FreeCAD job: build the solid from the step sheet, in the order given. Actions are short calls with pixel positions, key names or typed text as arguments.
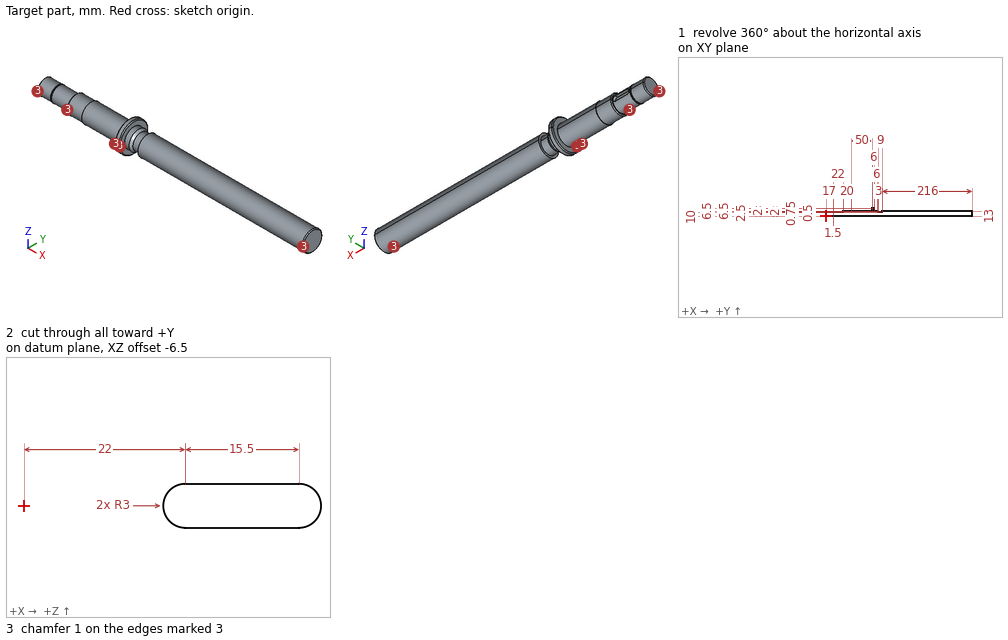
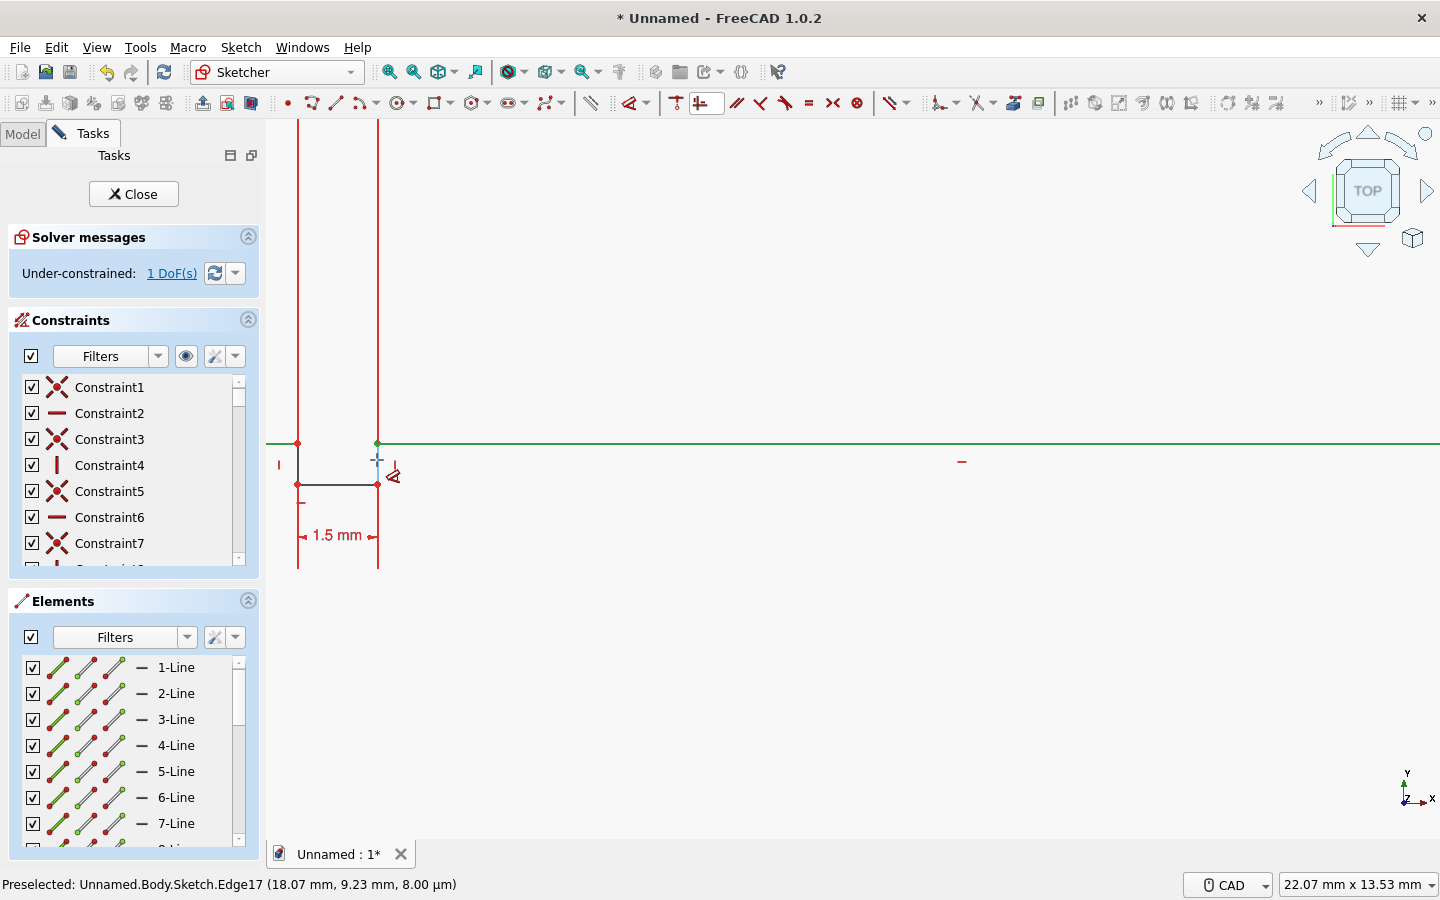
click(378, 460)
click(344, 464)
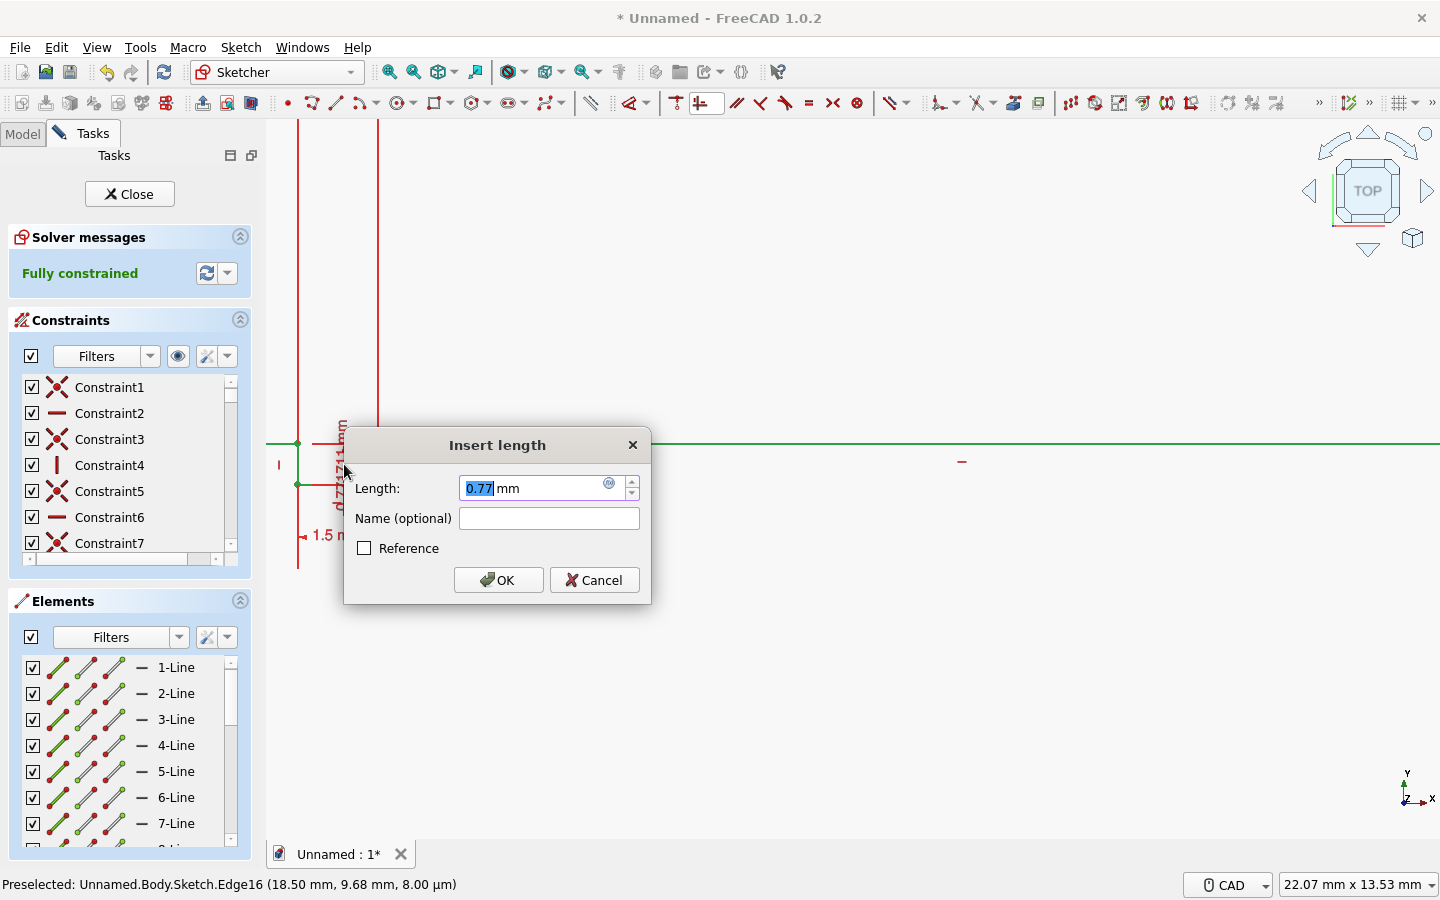
text(0.75)
key(Return)
key(Escape)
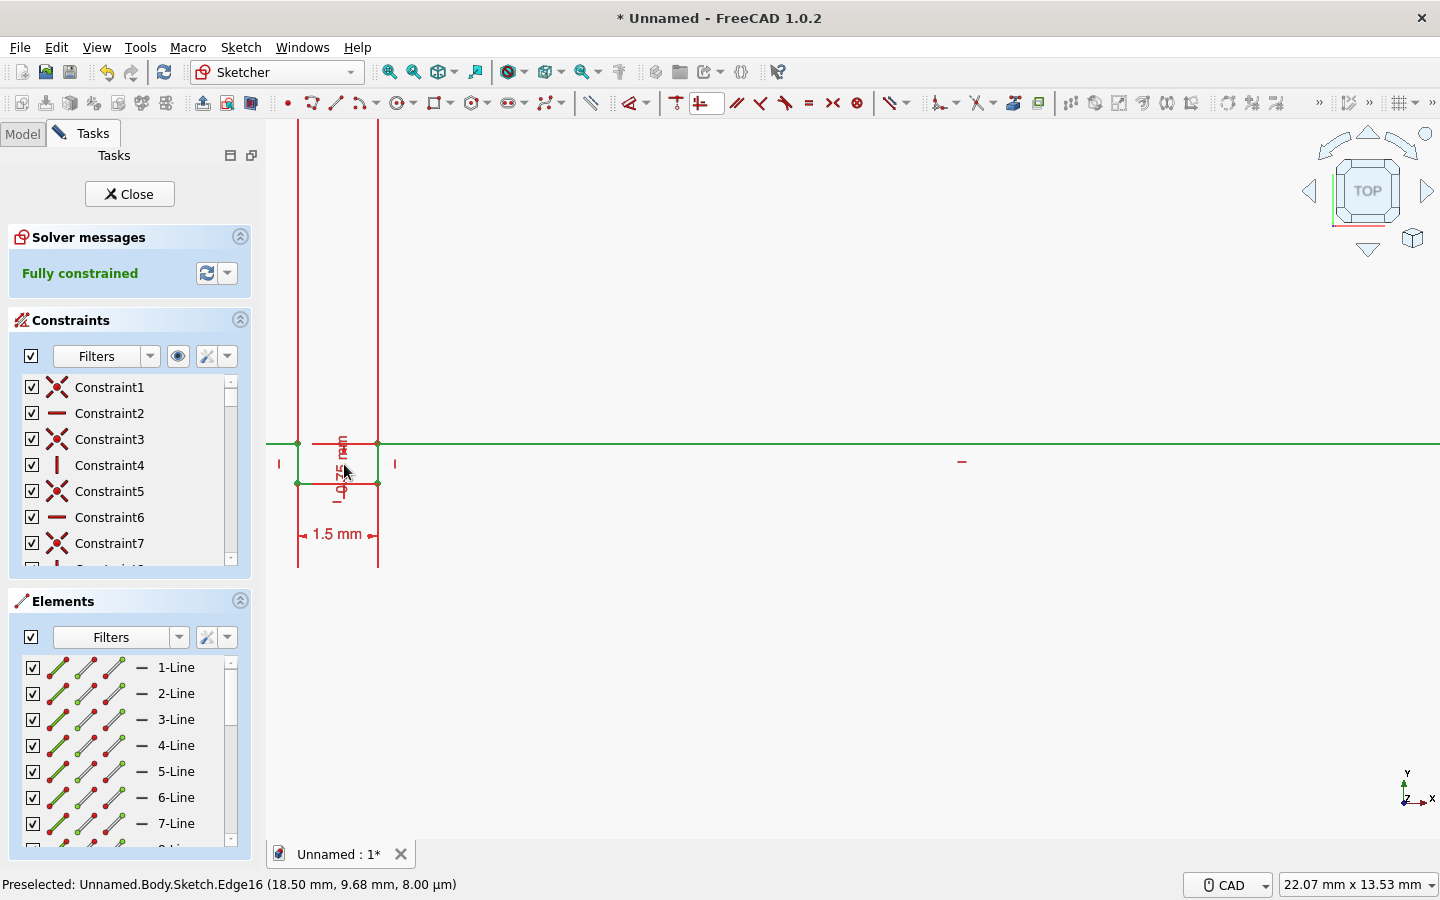
click(130, 194)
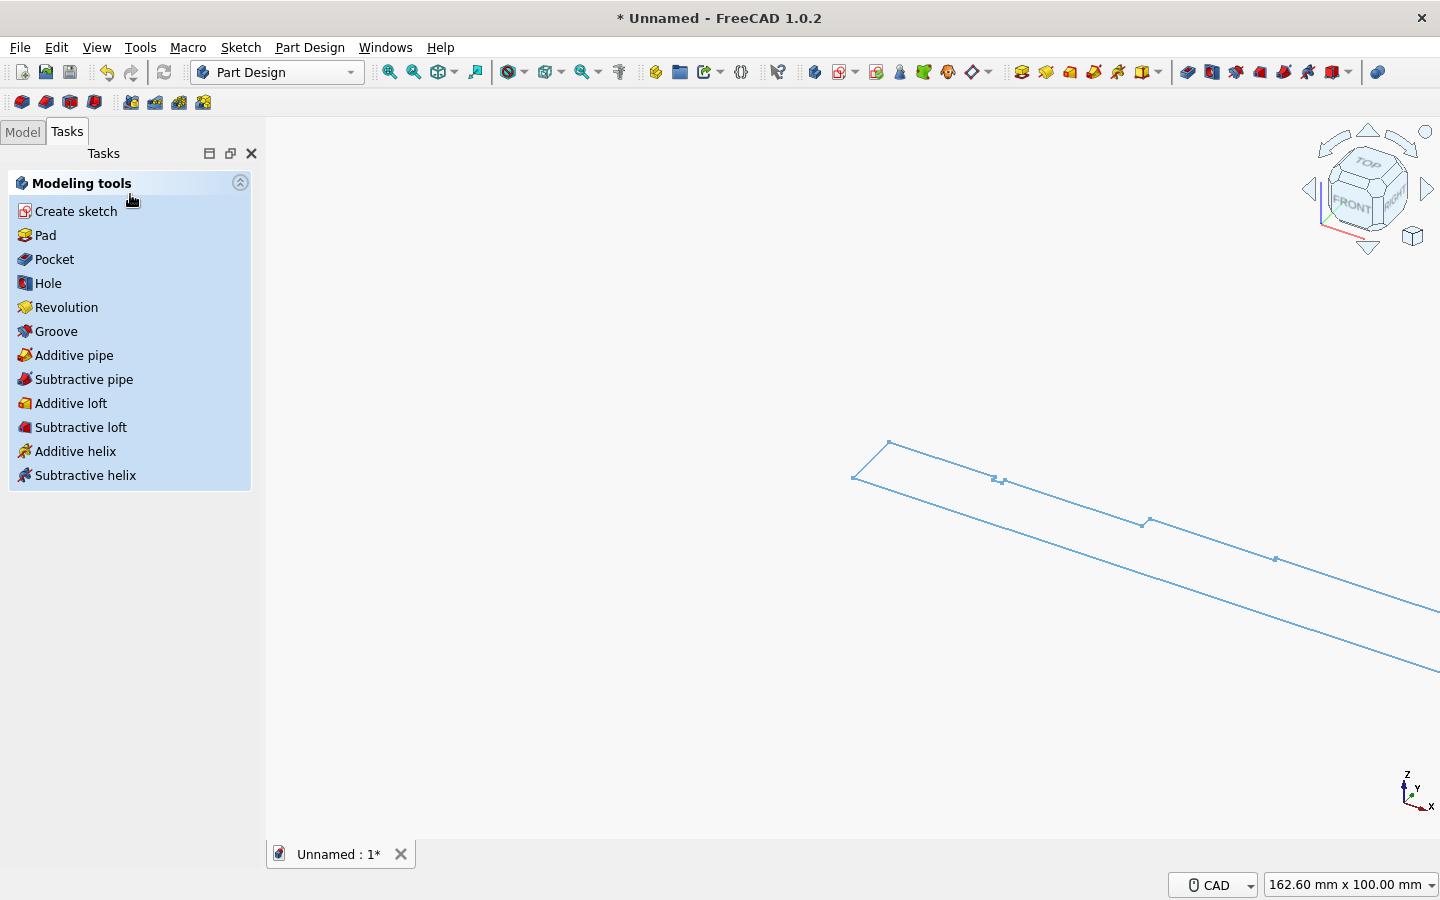
click(1046, 72)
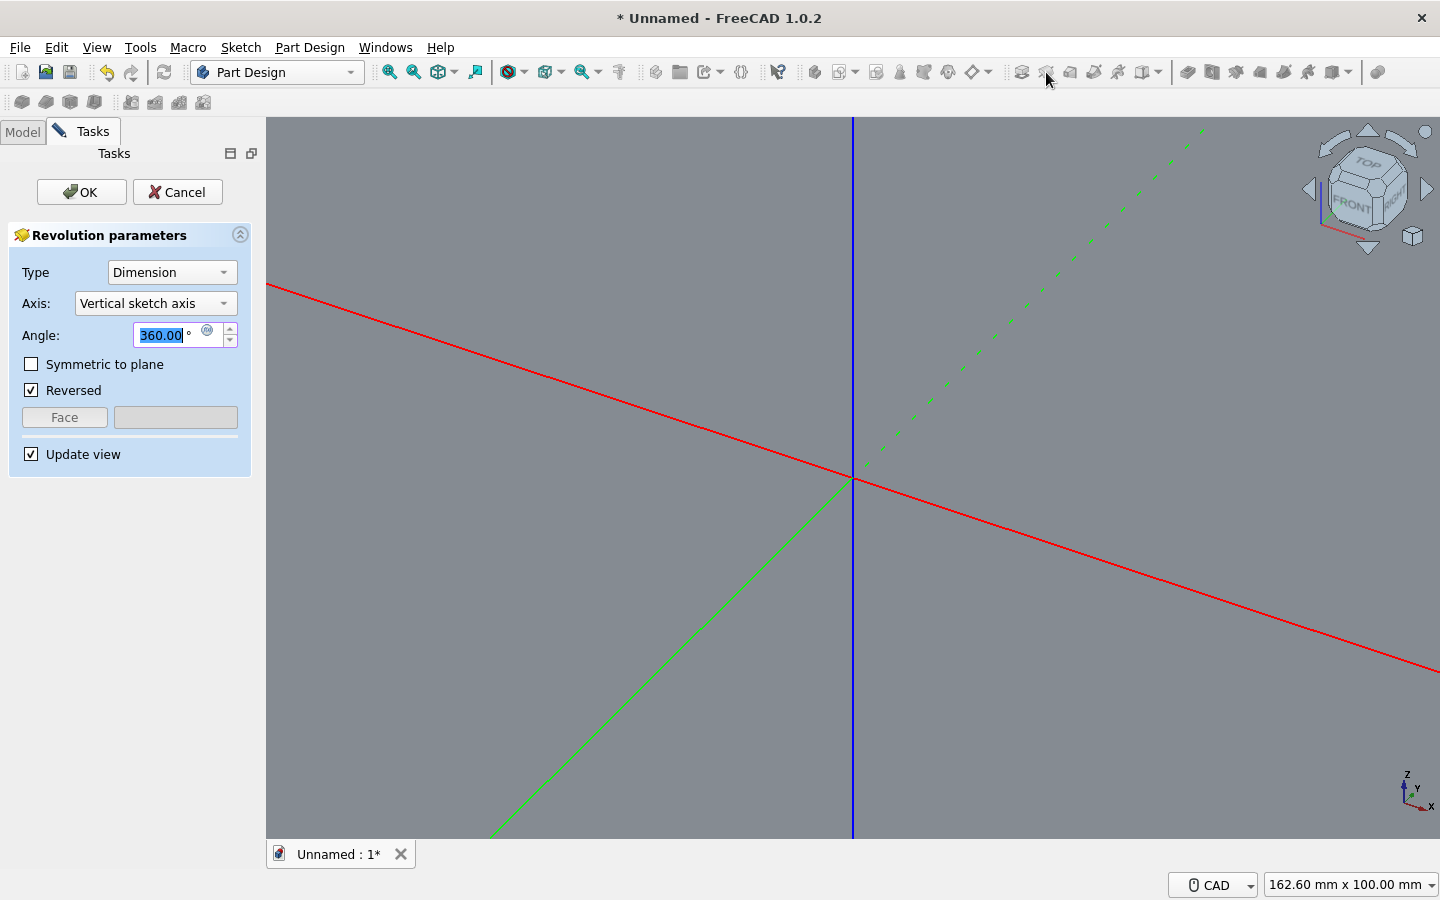
click(156, 304)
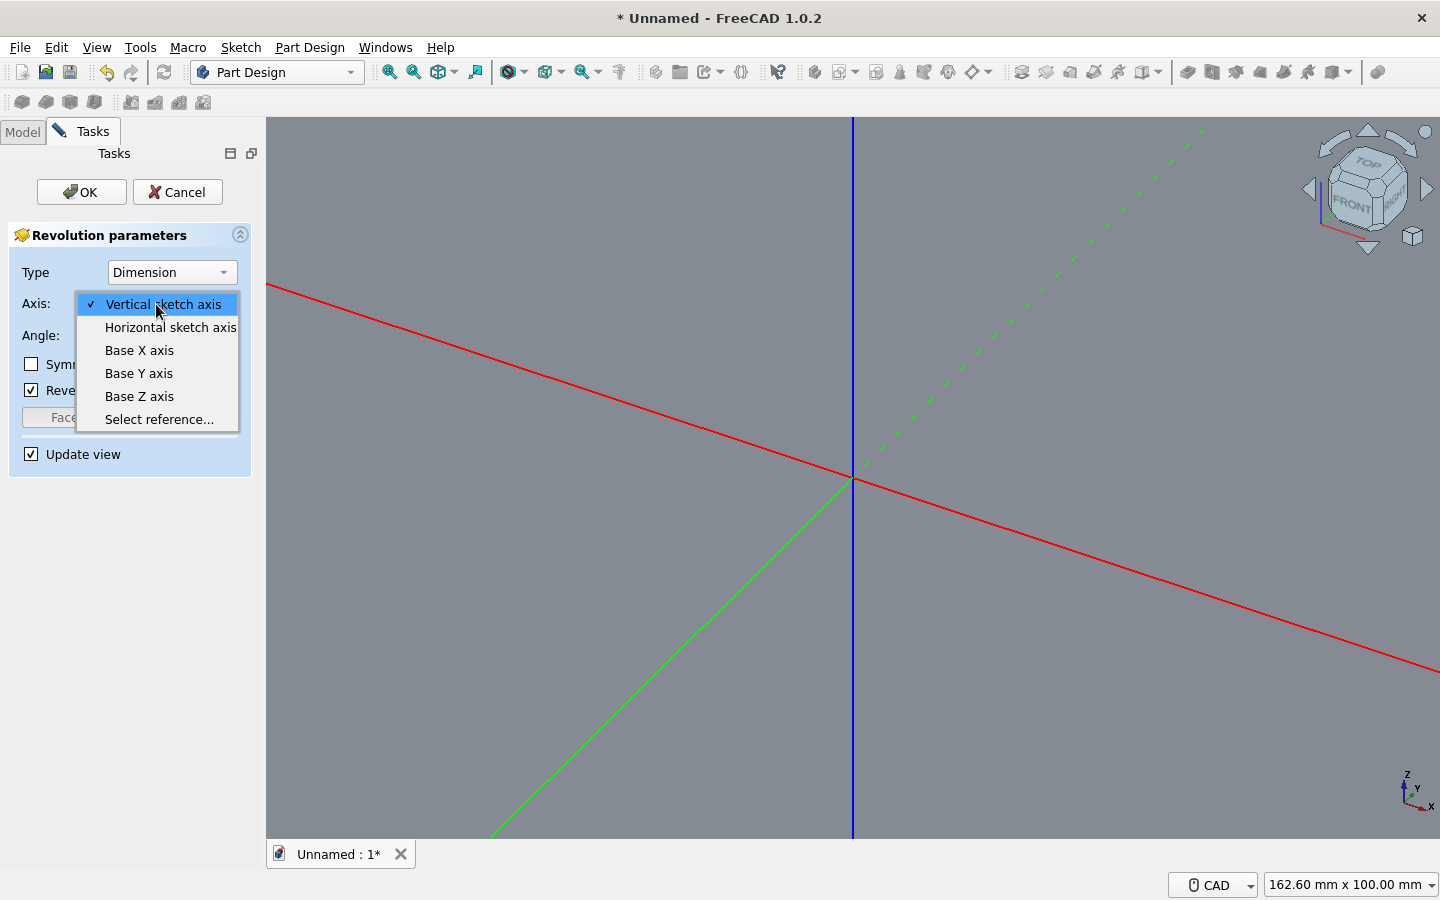
click(156, 328)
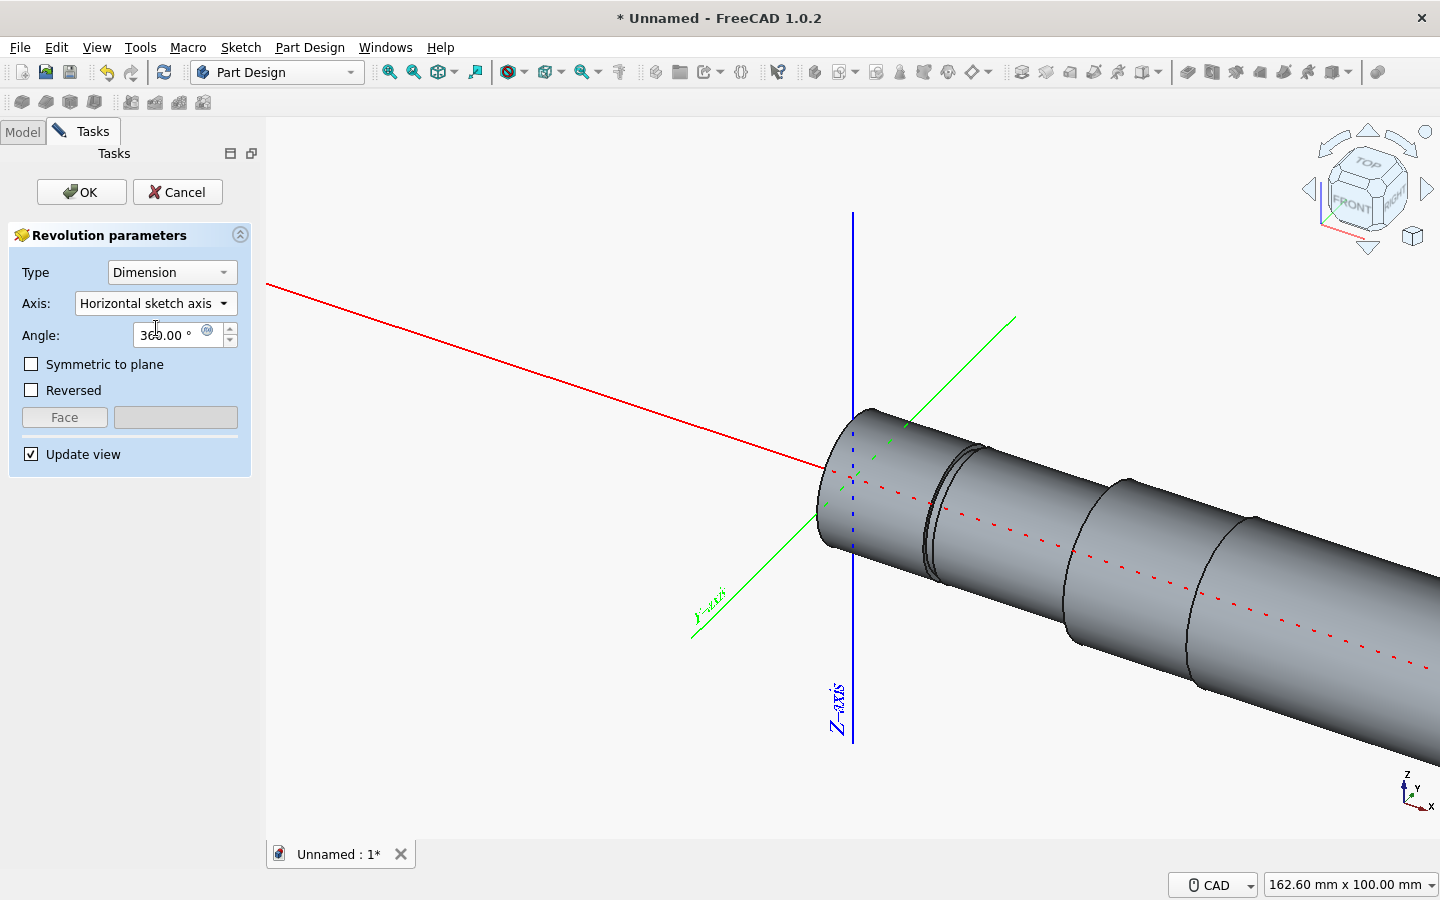
click(82, 192)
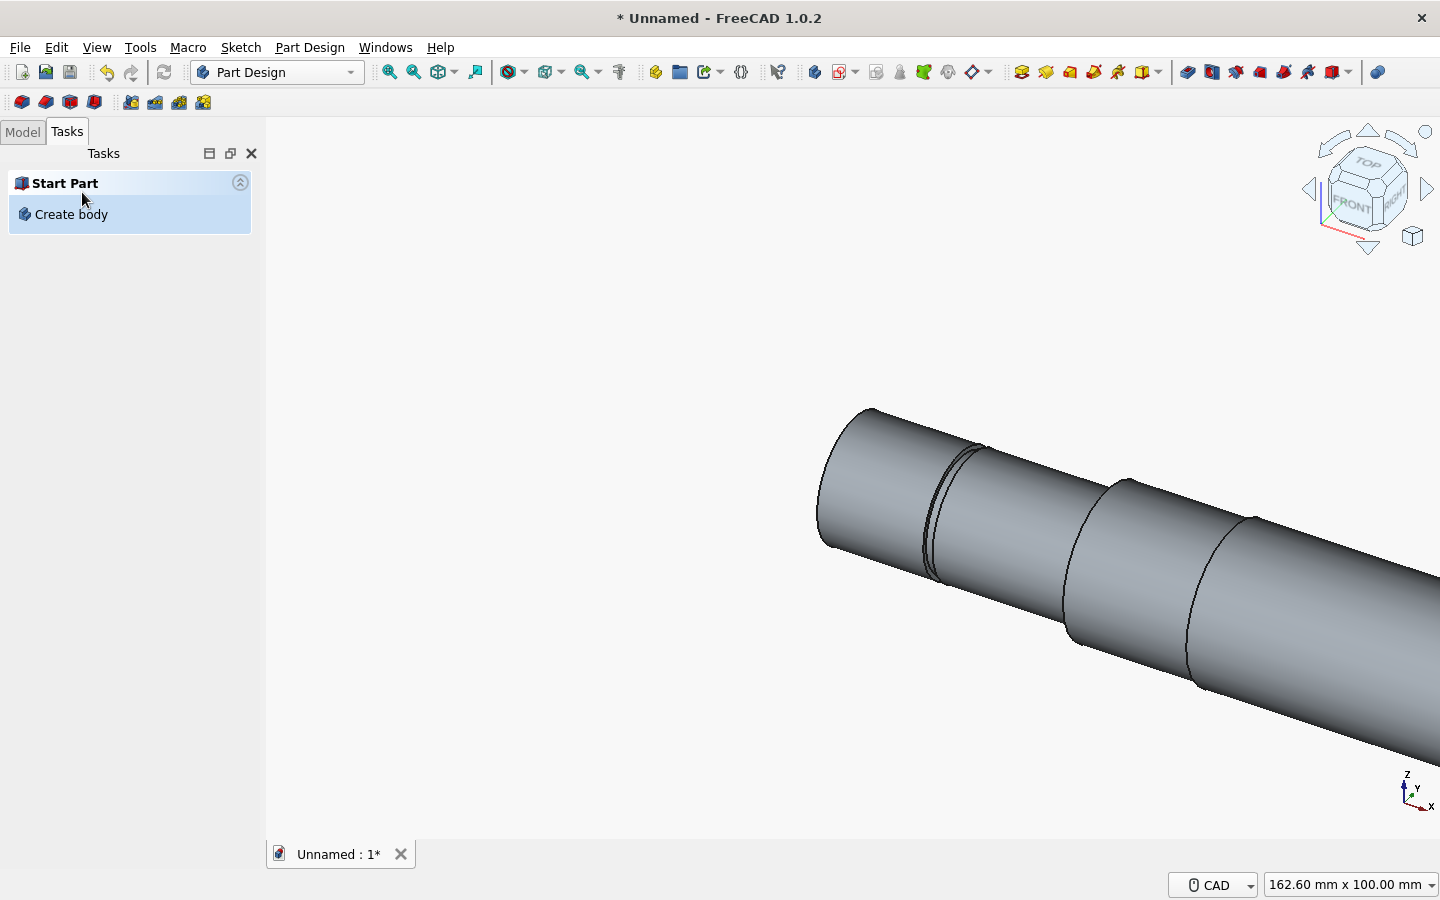
click(390, 72)